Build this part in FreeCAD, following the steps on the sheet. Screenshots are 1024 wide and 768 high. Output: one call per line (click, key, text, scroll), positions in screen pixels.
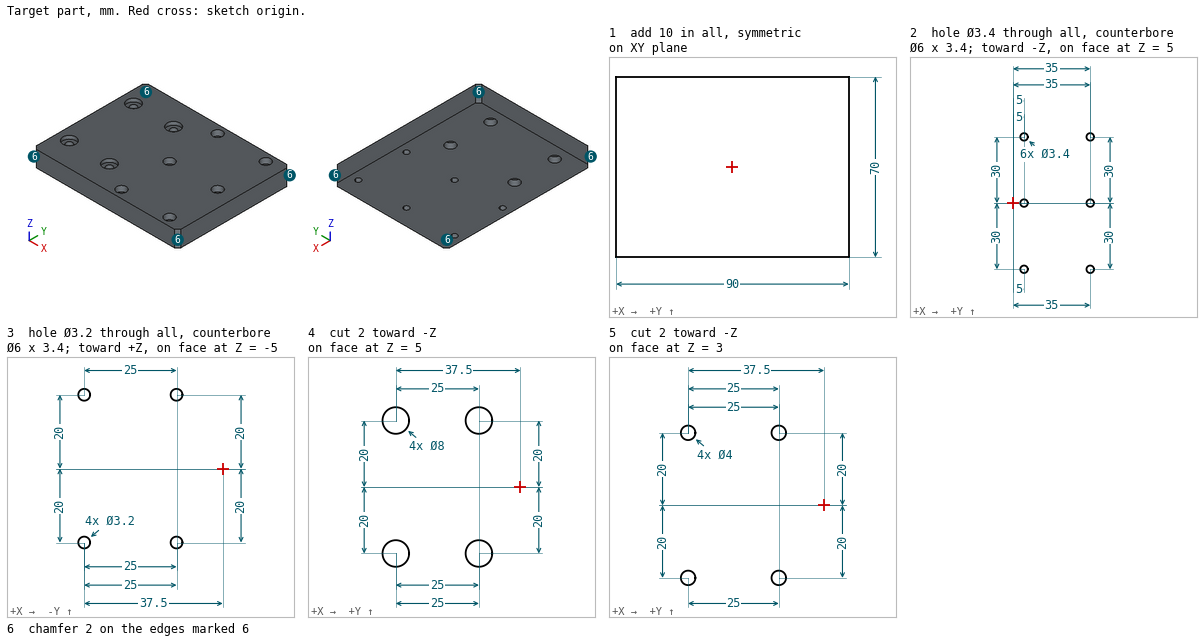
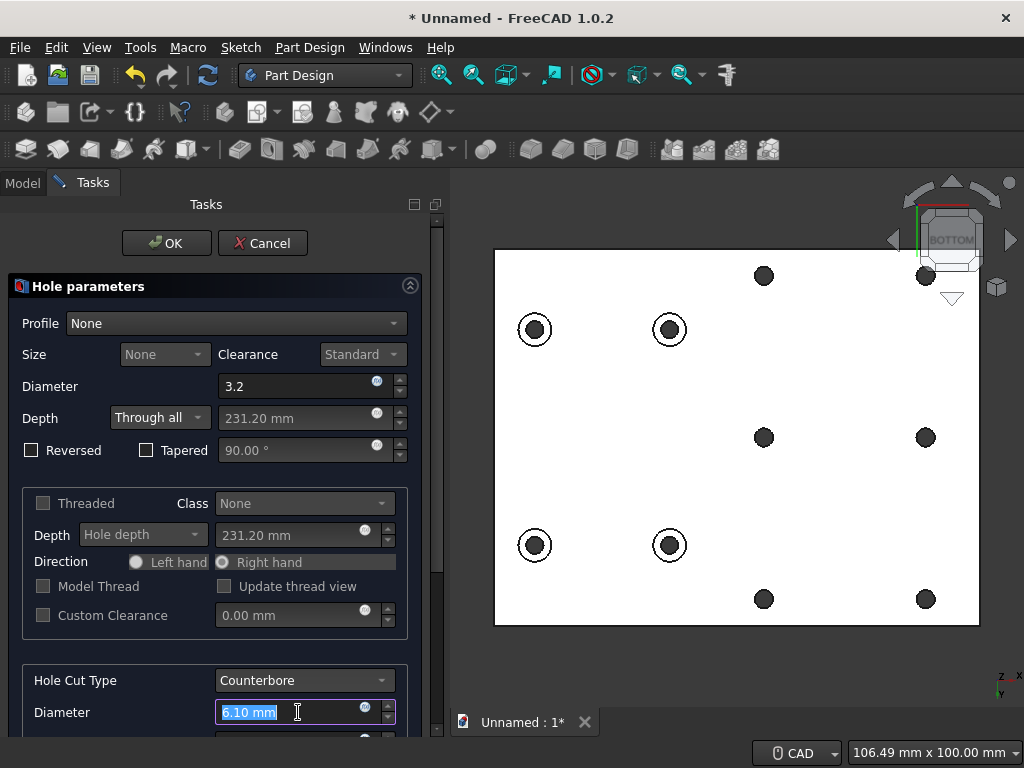
text(6)
key(Tab)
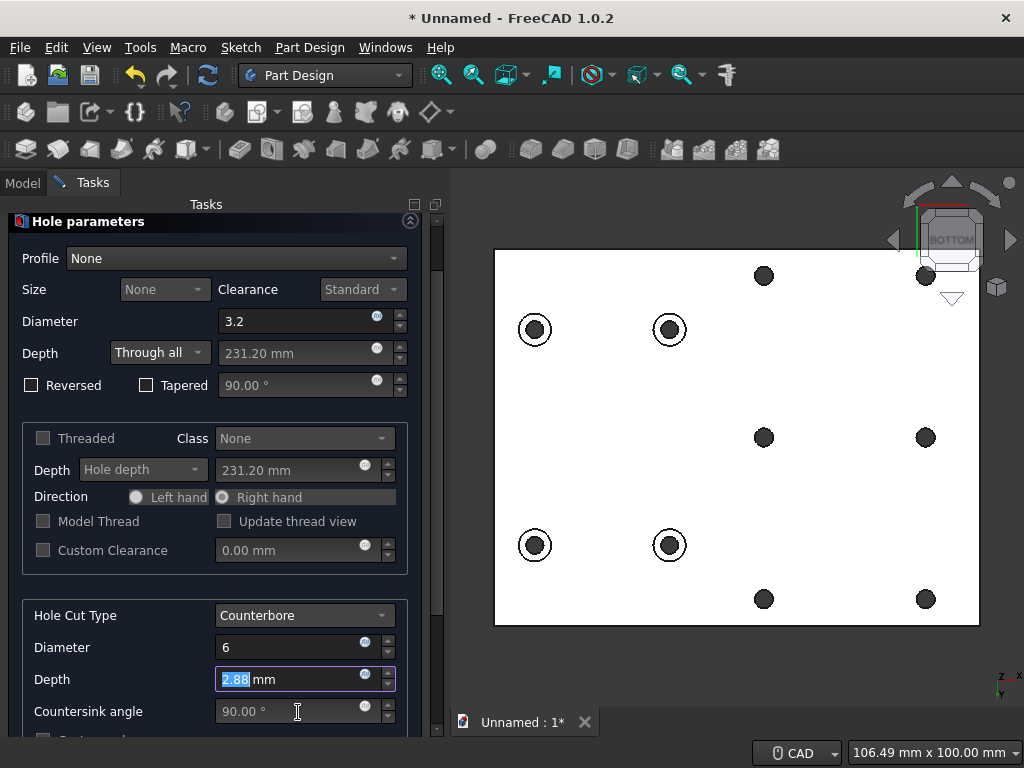
text(3.4)
key(Tab)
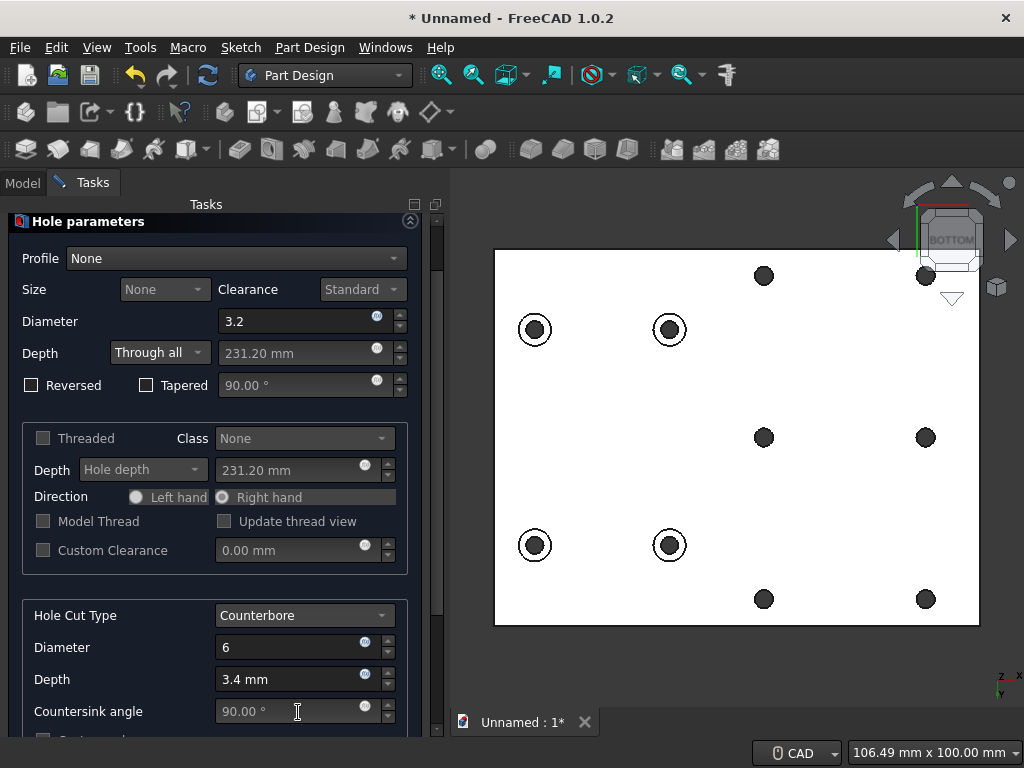
scroll(437, 475, up, 2)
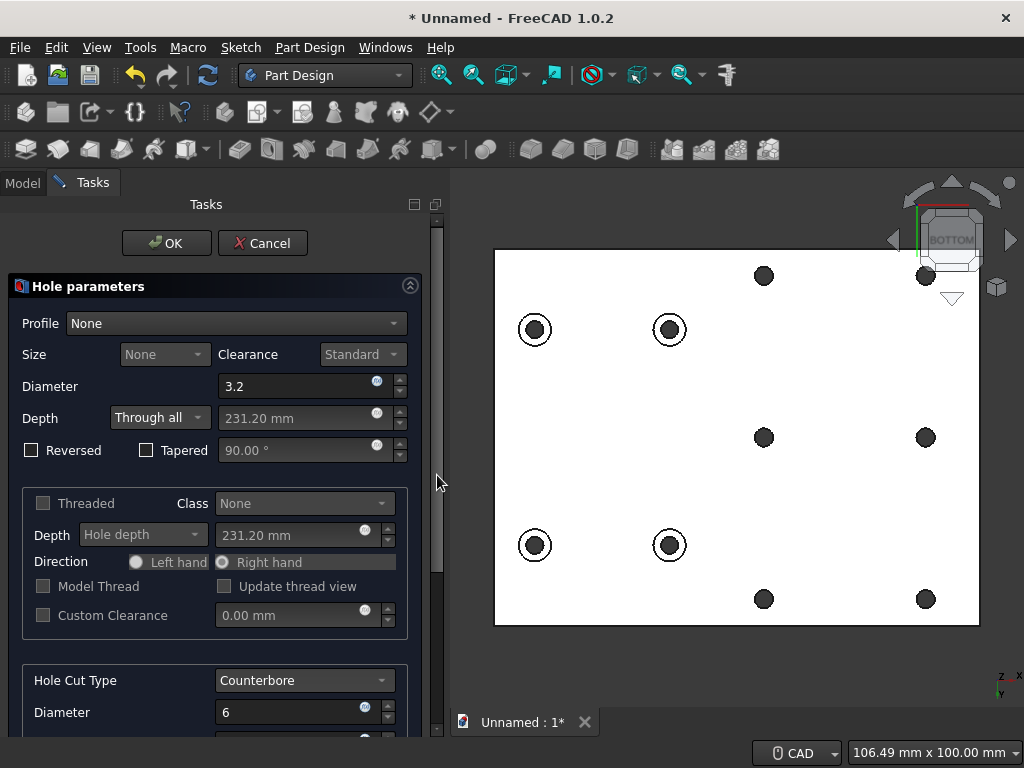
click(167, 243)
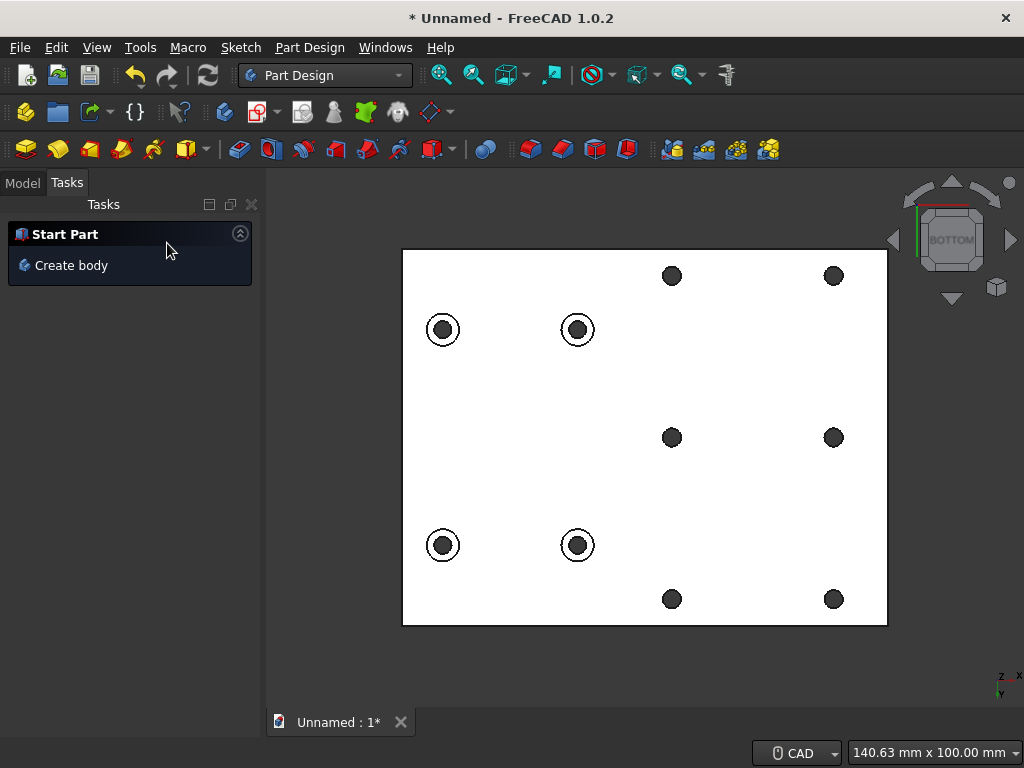
key(0)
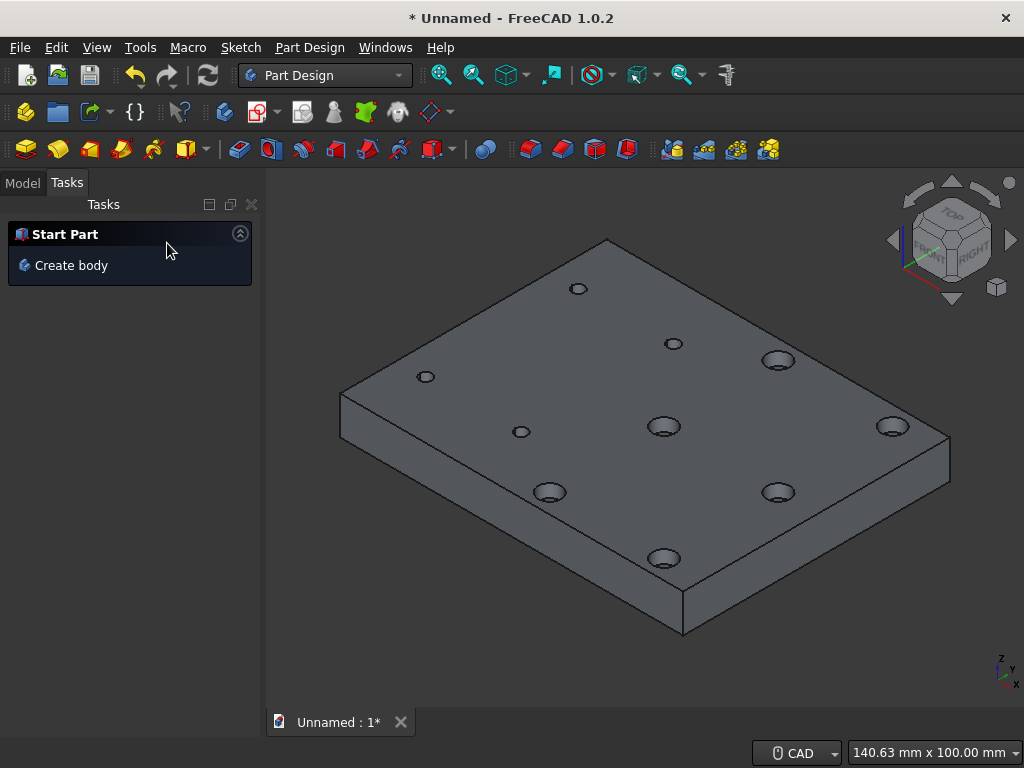
click(547, 358)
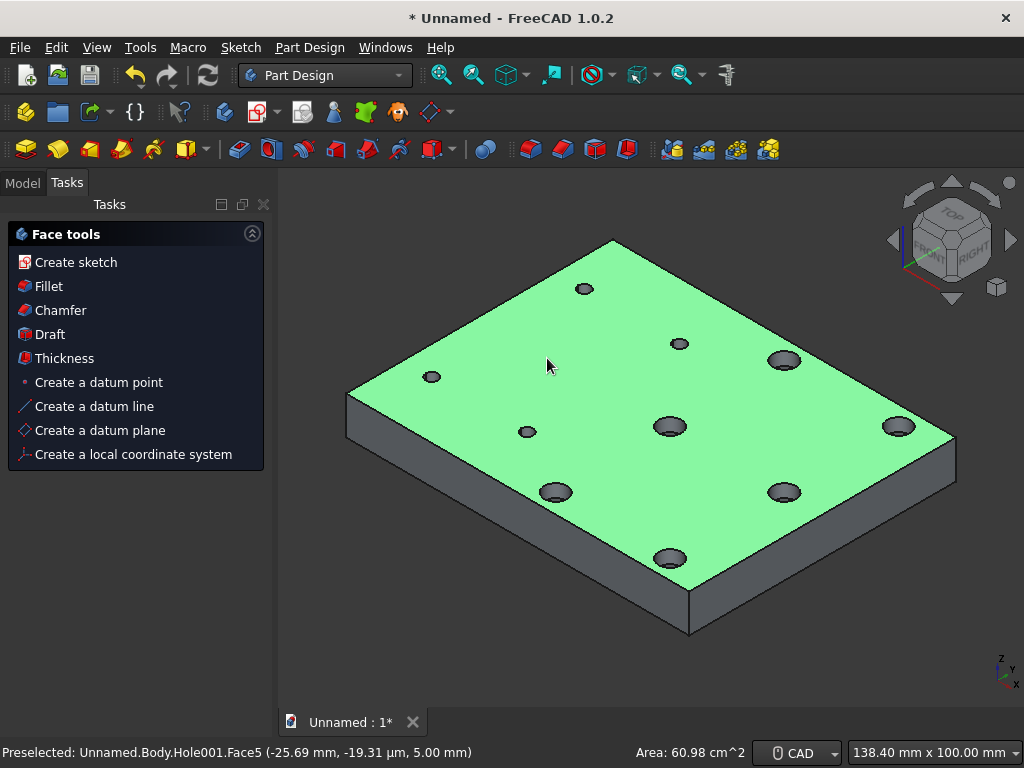
click(258, 112)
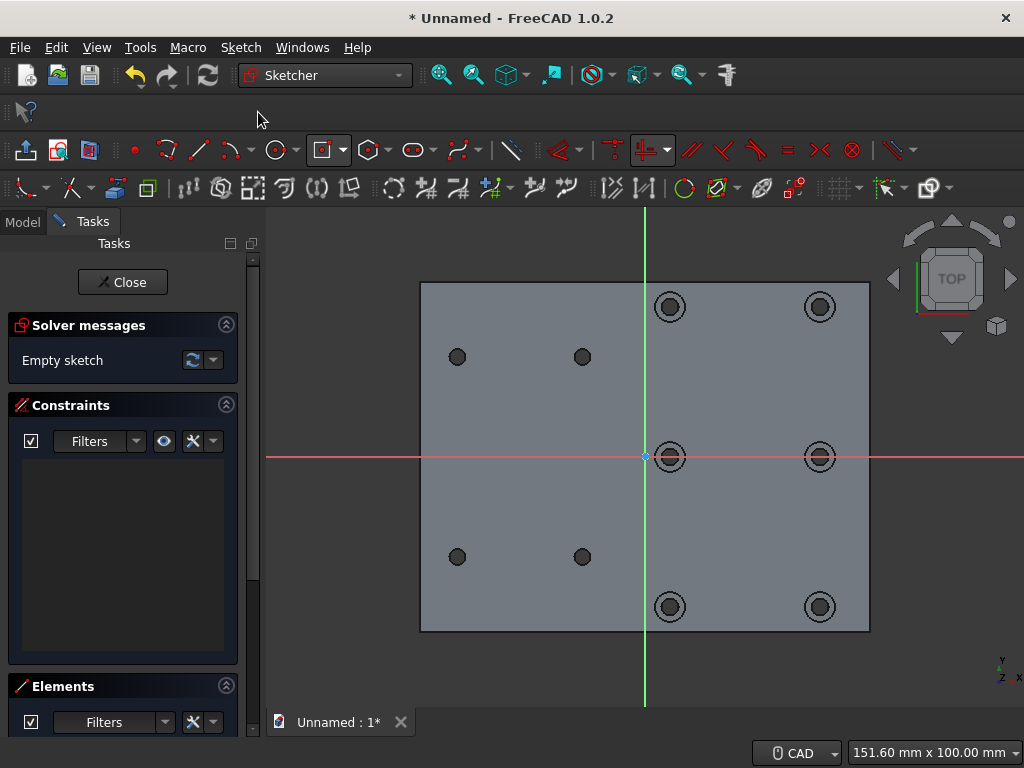
click(276, 150)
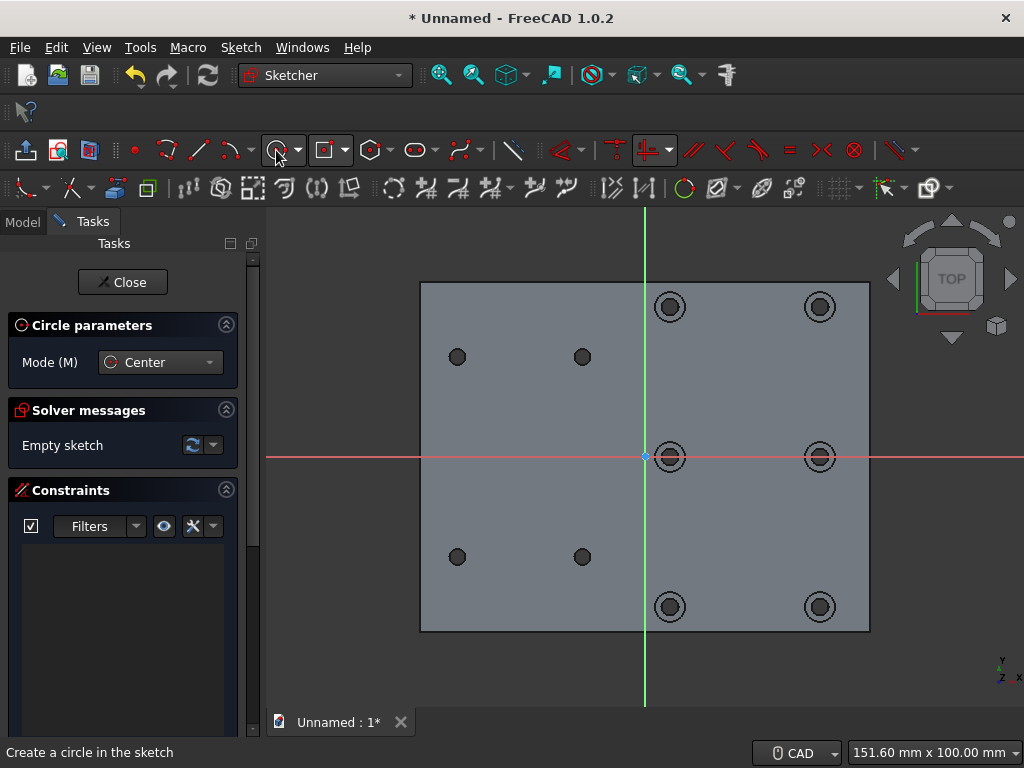
click(457, 357)
click(472, 343)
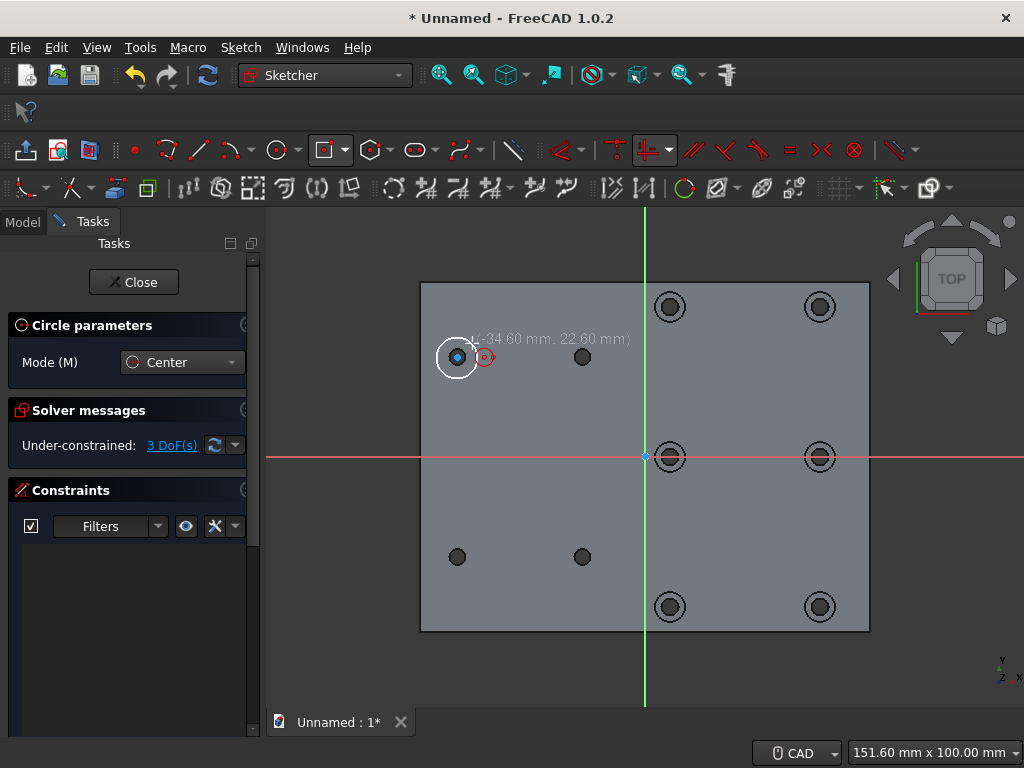
click(582, 357)
click(597, 343)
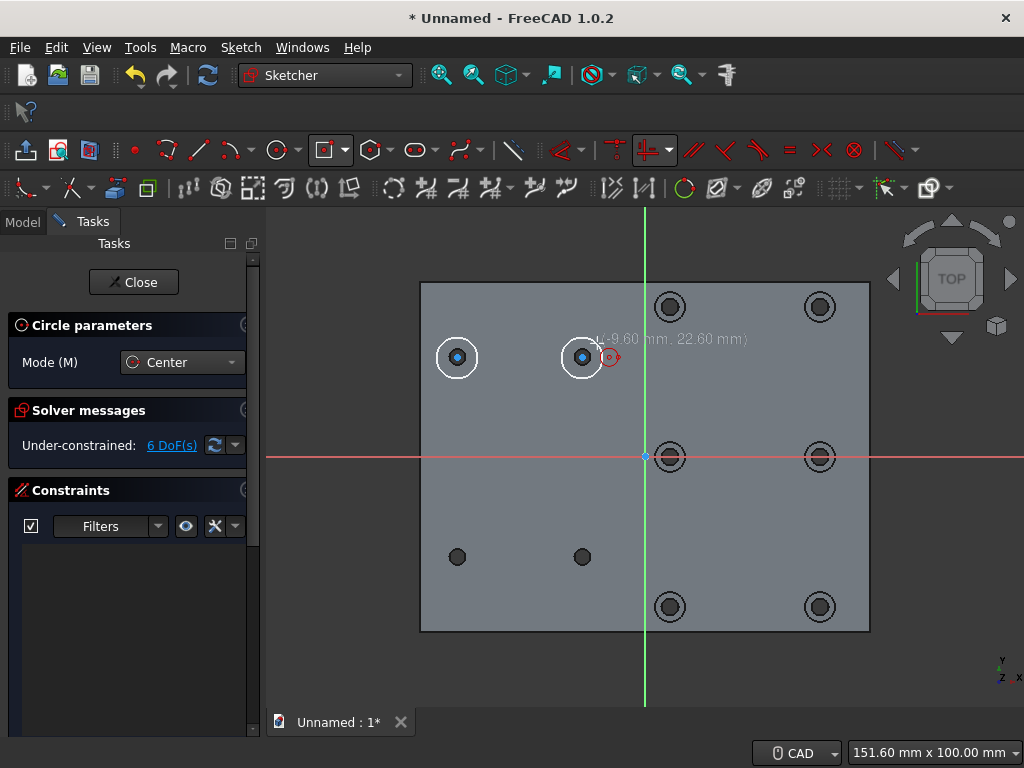
click(457, 557)
click(472, 543)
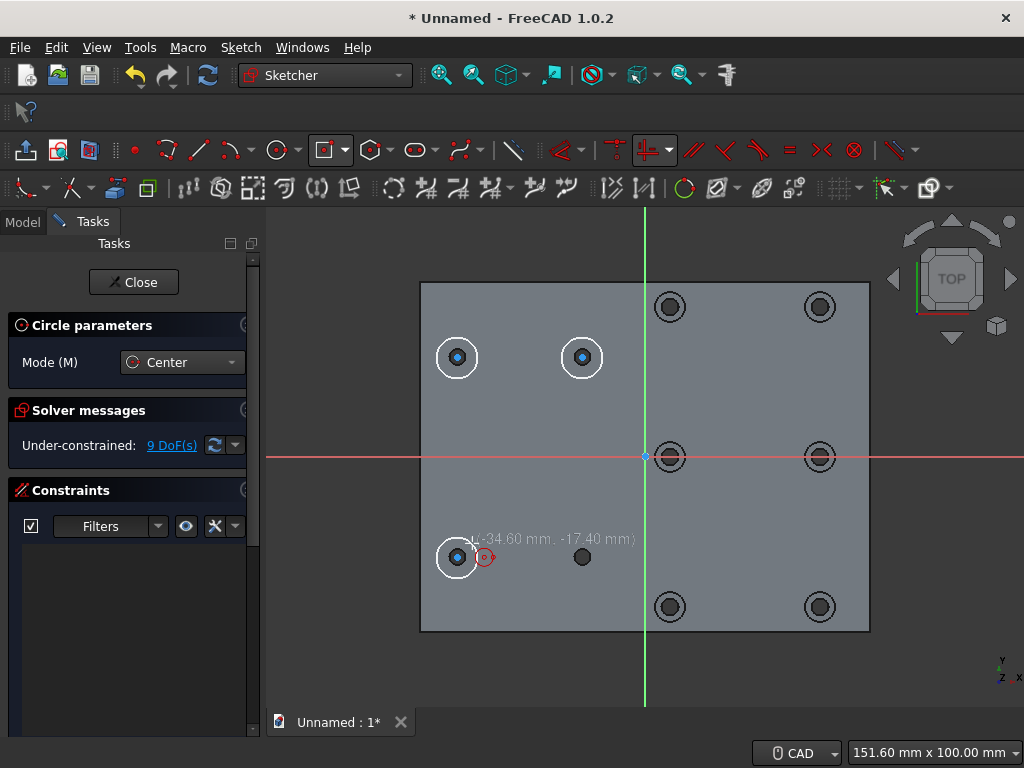
click(582, 557)
click(597, 543)
key(Escape)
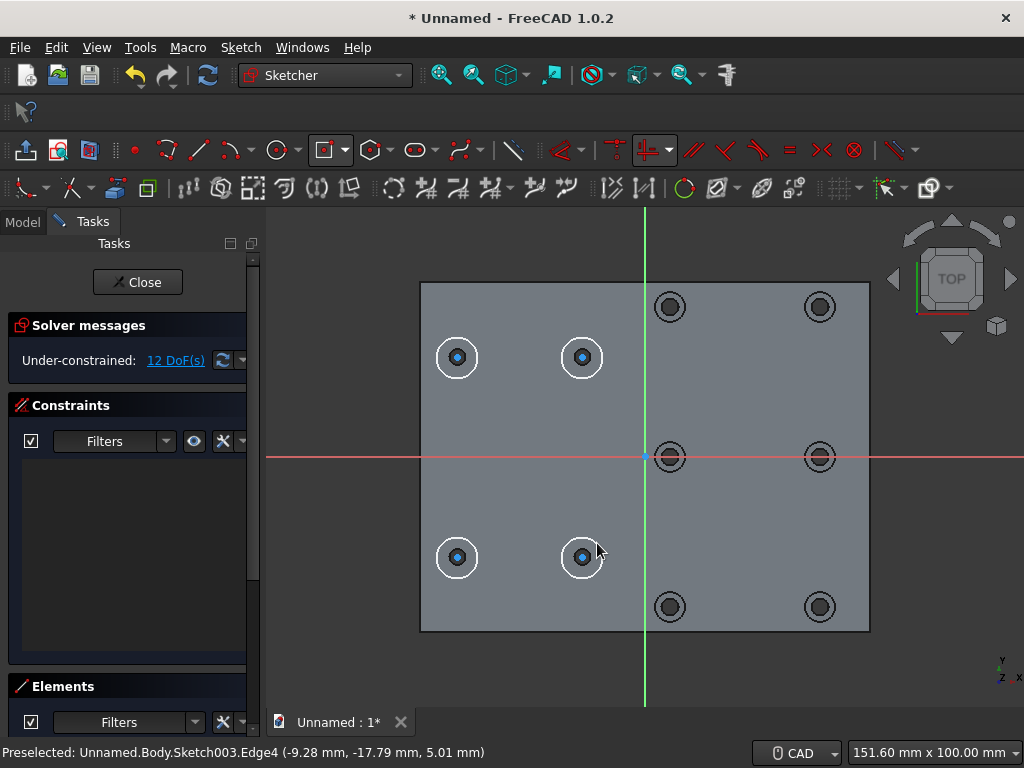
click(471, 343)